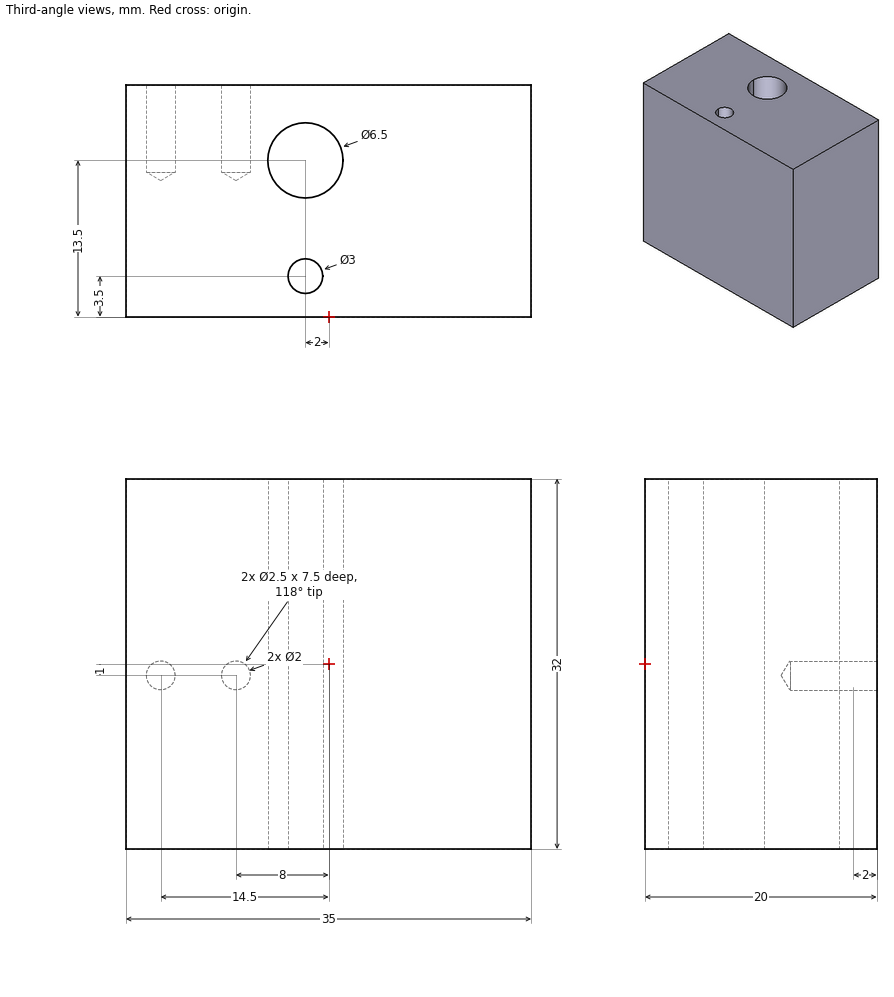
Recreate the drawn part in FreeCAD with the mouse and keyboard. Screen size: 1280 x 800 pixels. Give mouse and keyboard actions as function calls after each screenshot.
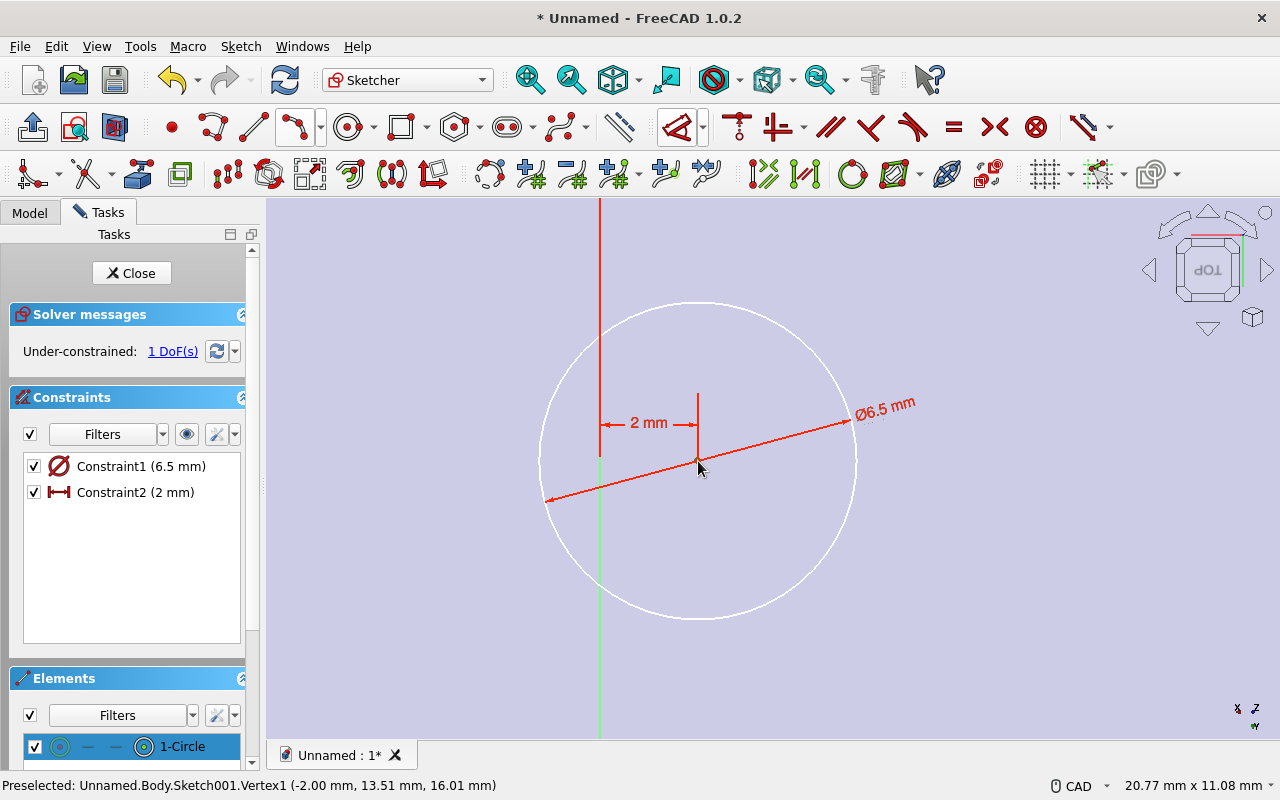
click(702, 128)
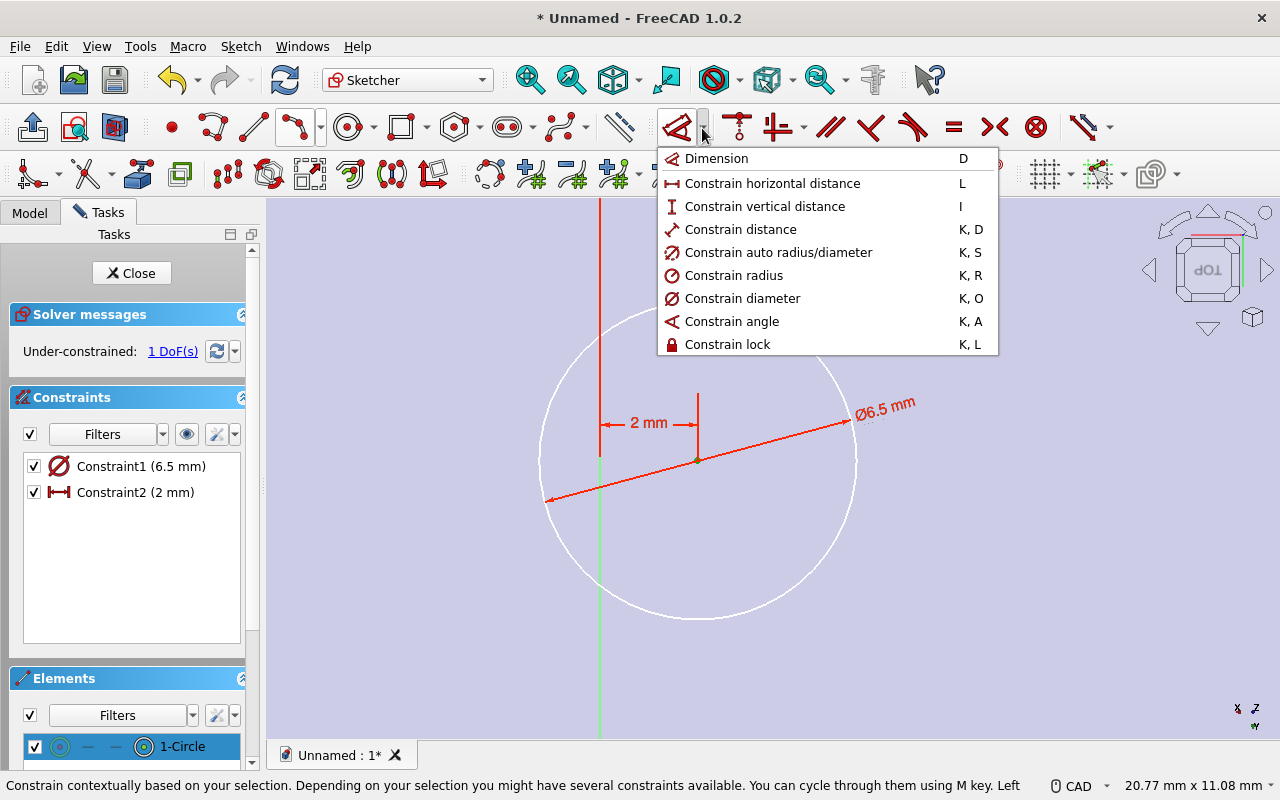
click(828, 206)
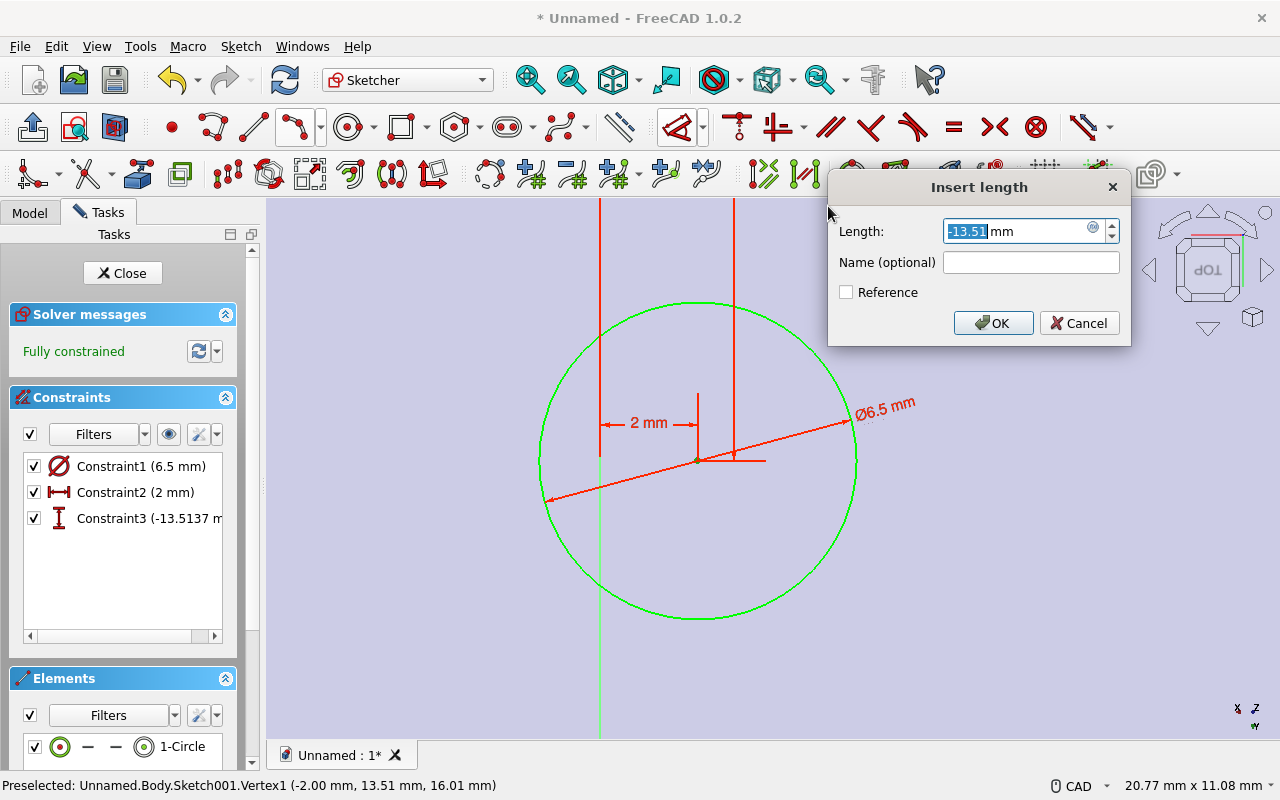
text(-13.5)
key(Return)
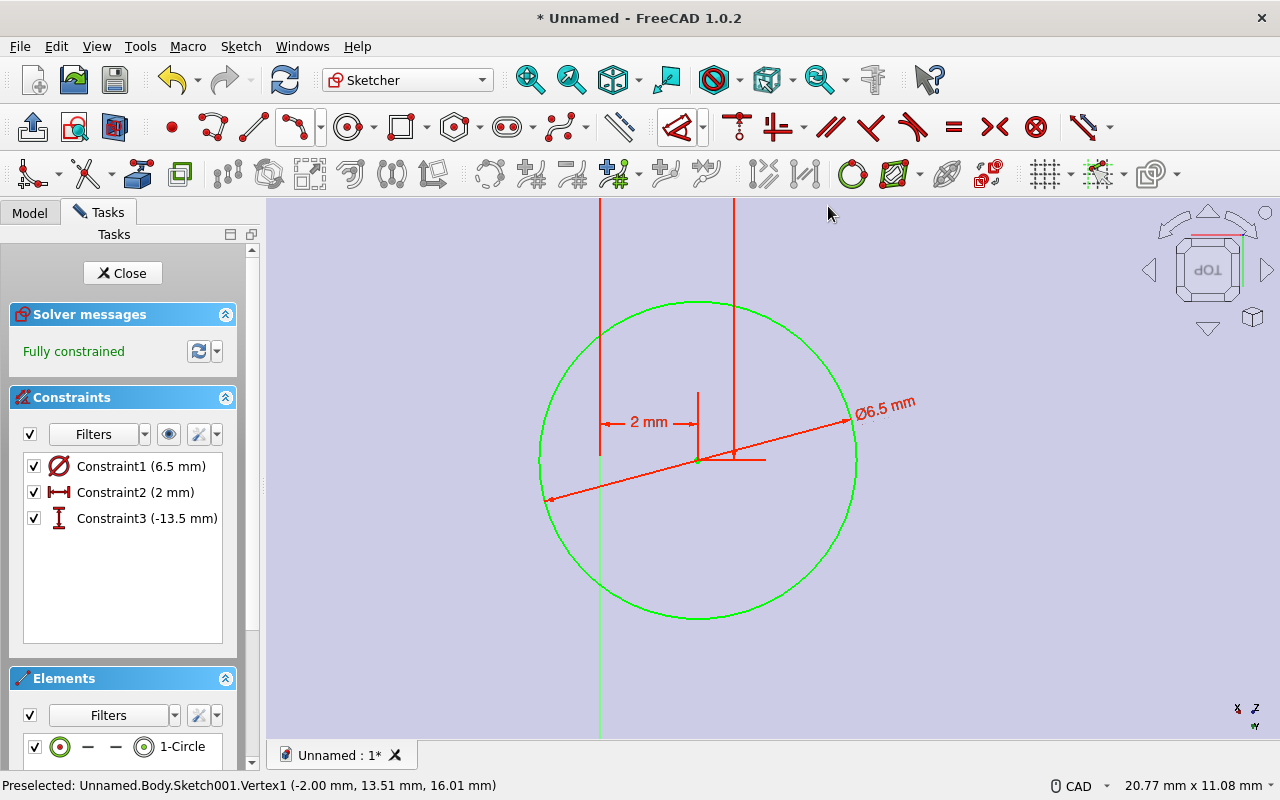
click(123, 273)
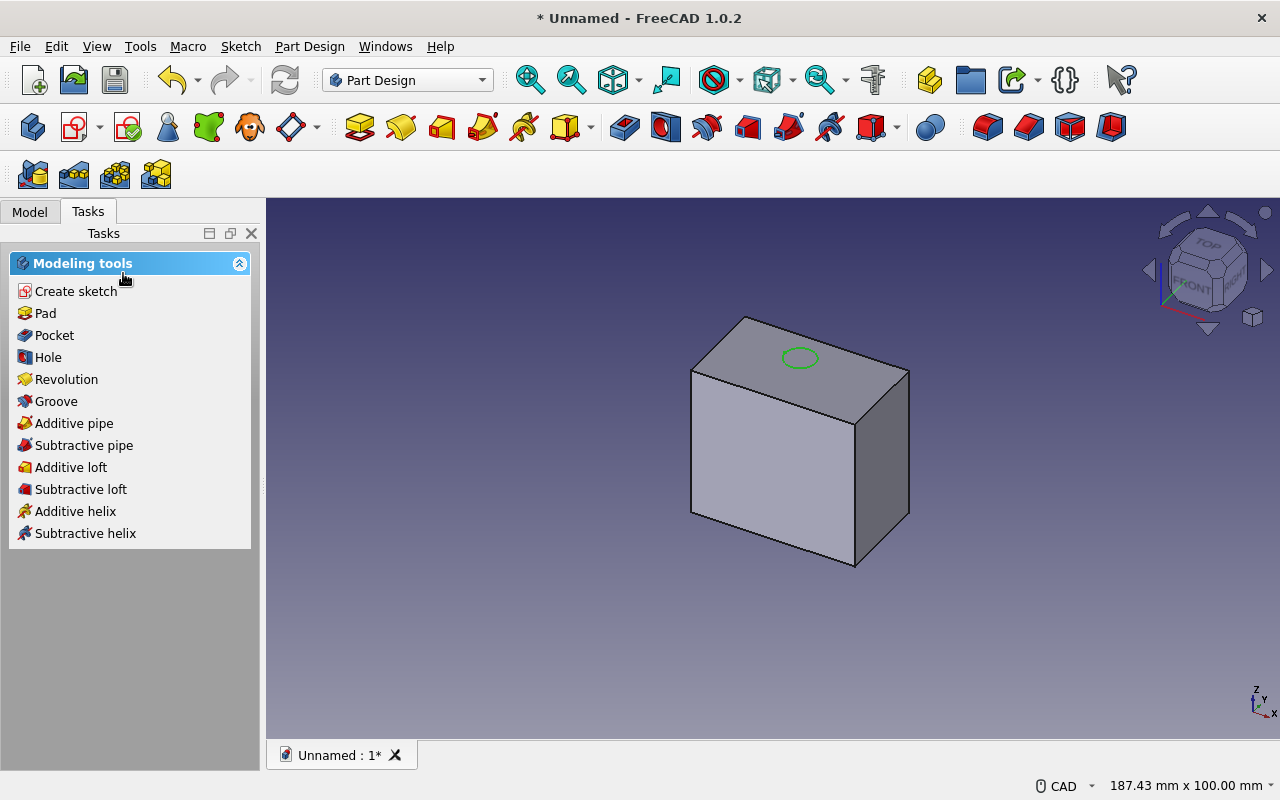
click(625, 128)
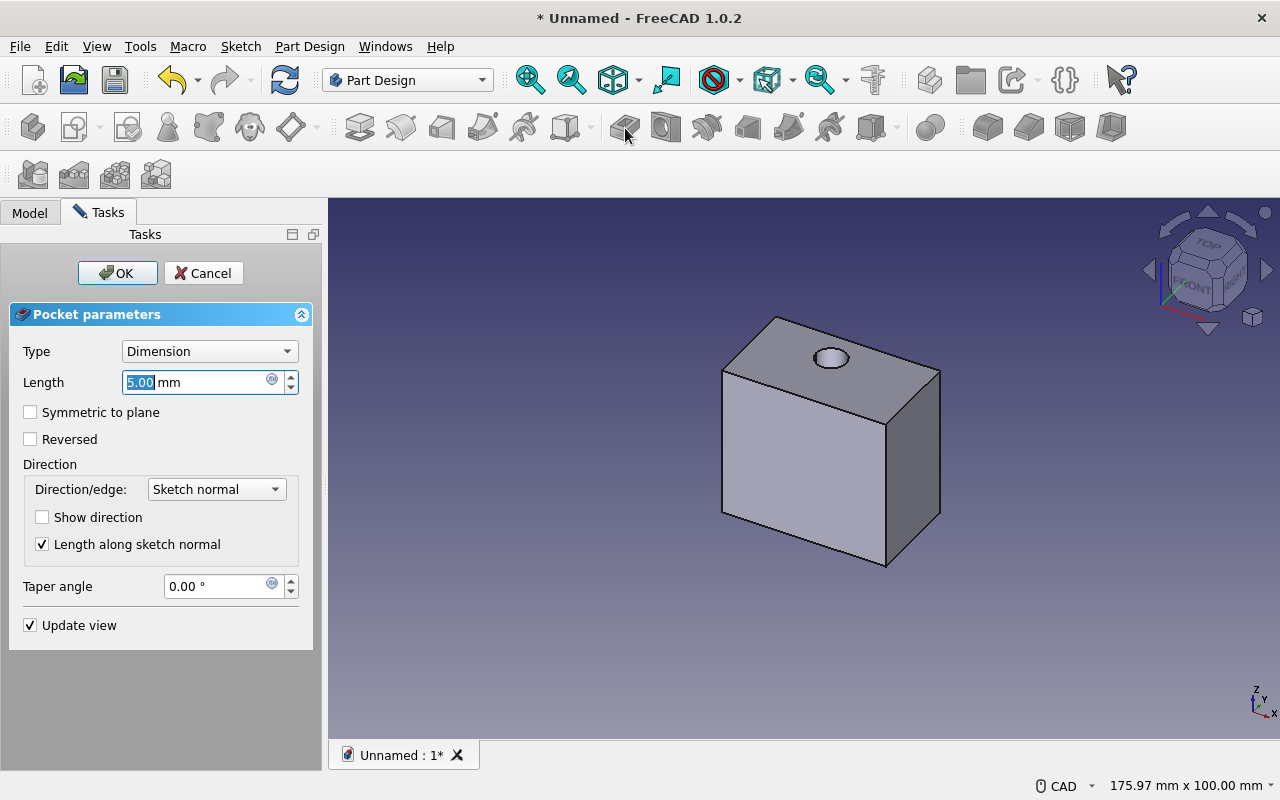
click(210, 352)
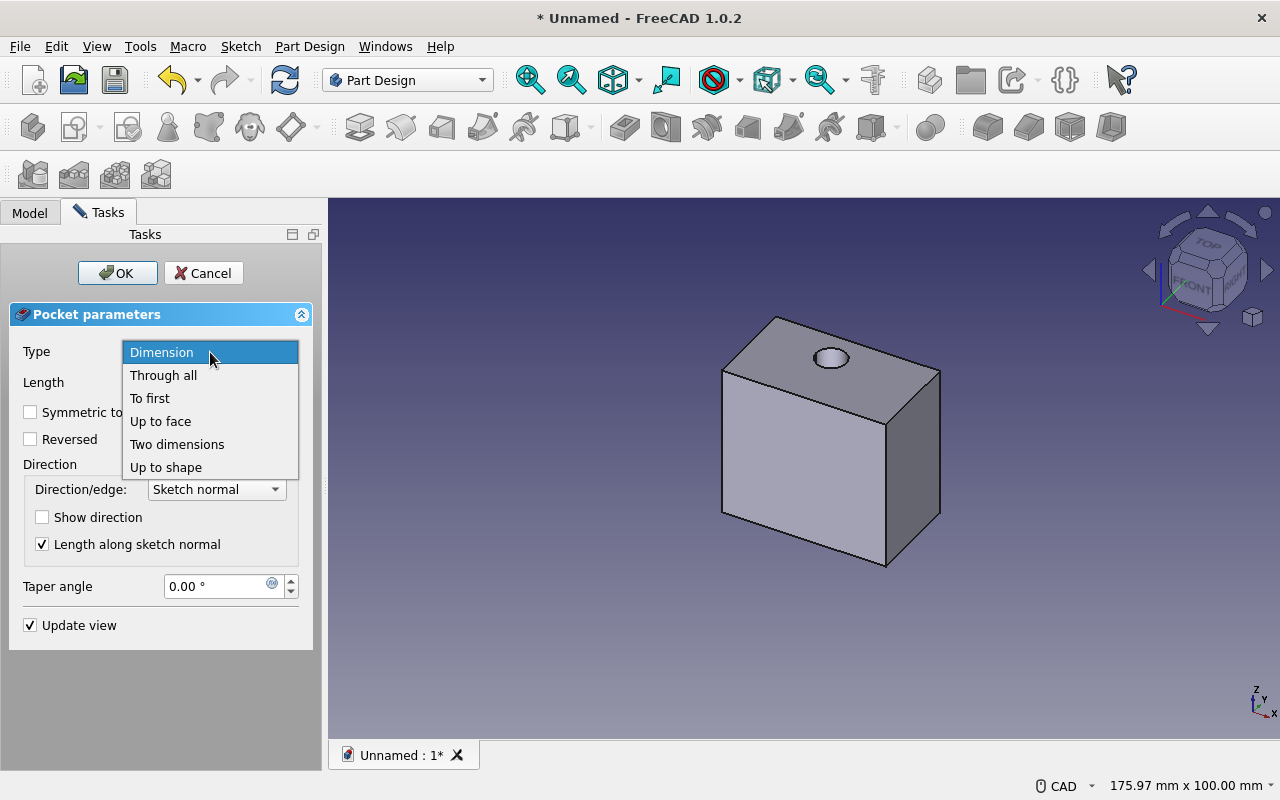
click(208, 398)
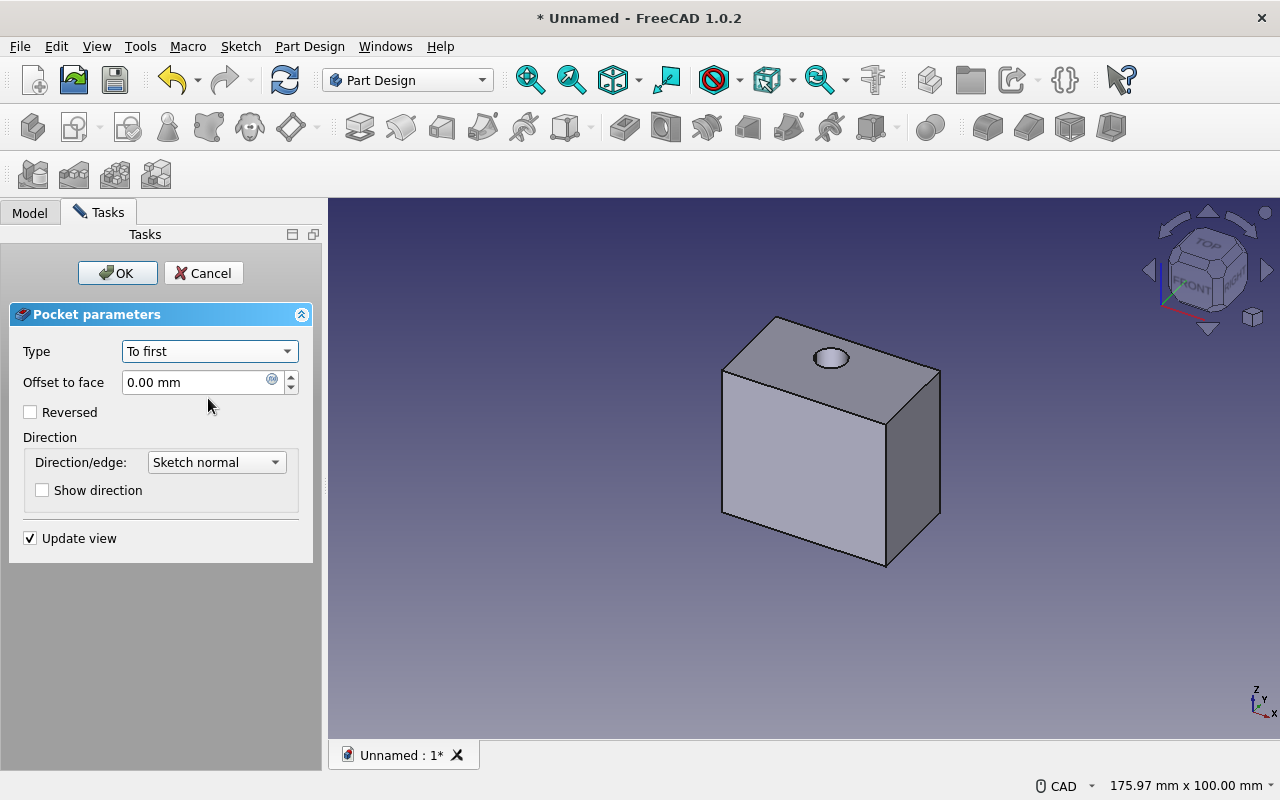
click(118, 273)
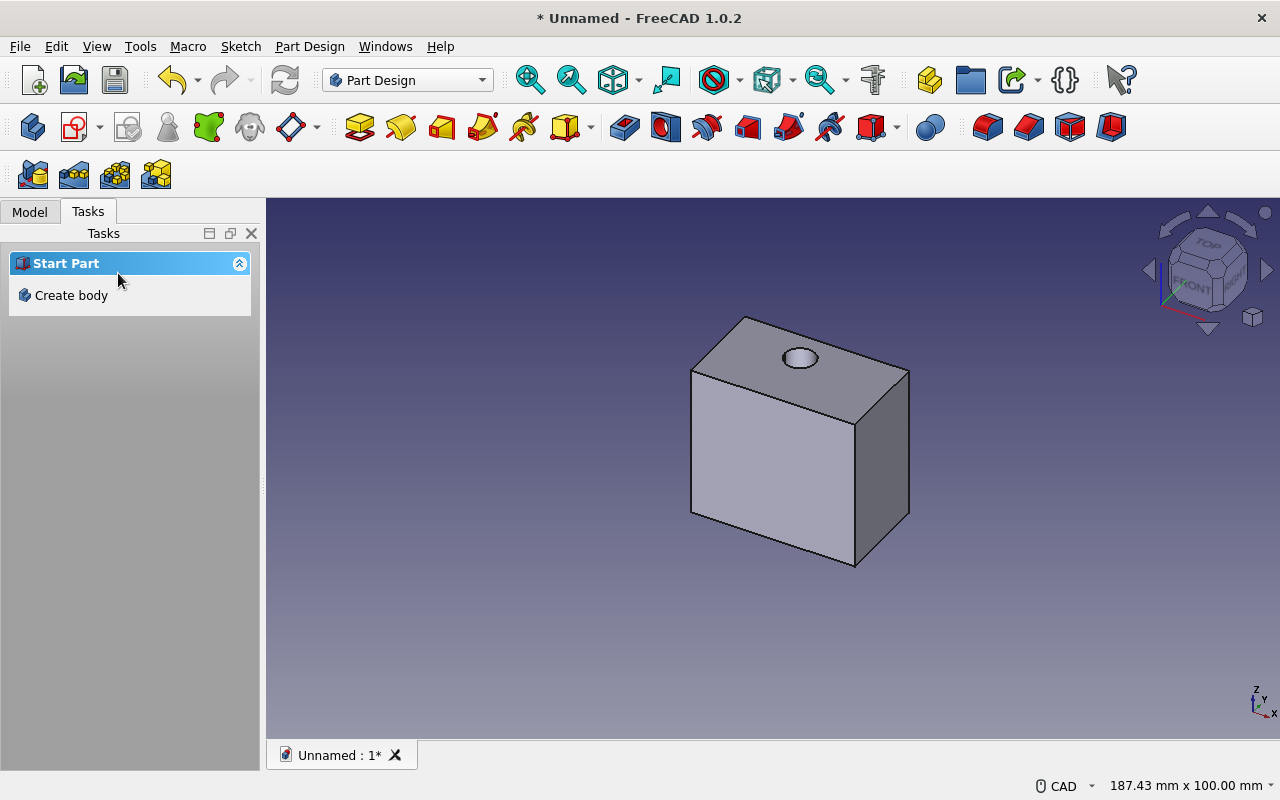
click(847, 385)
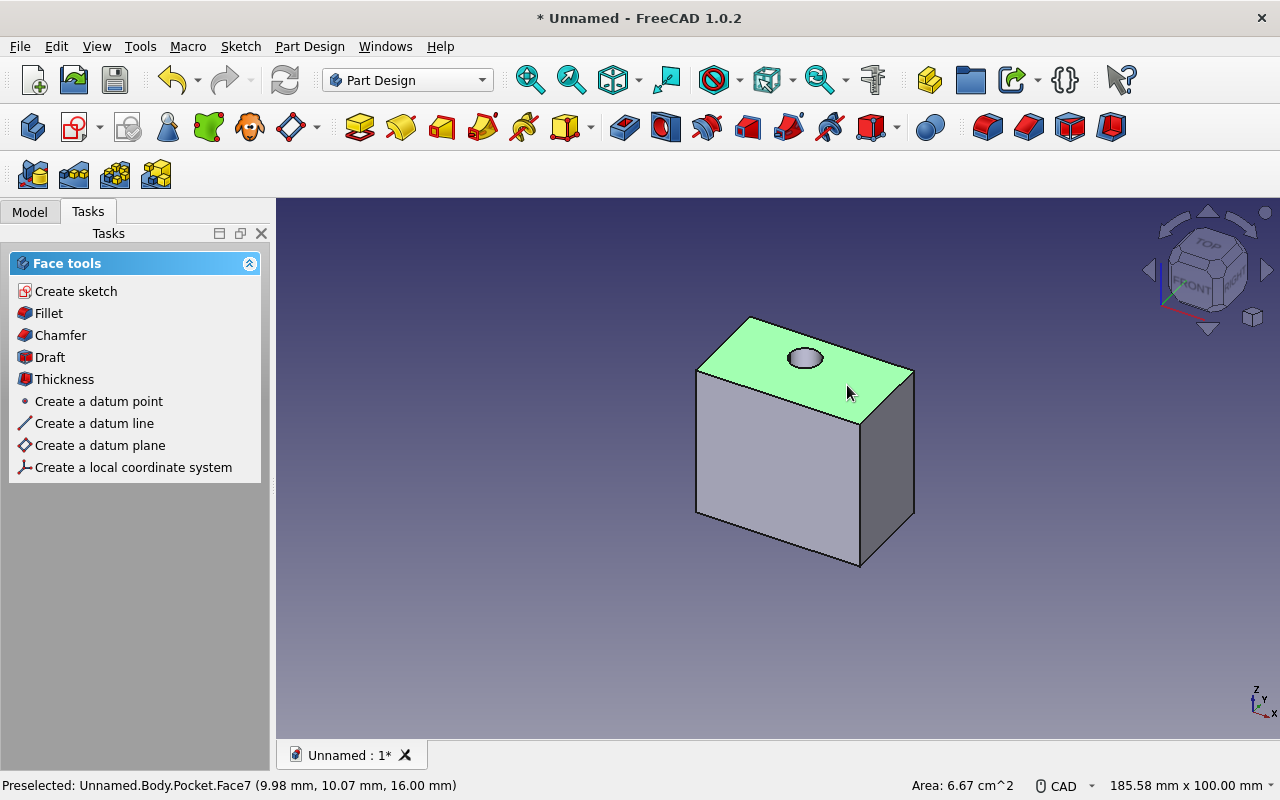
click(74, 128)